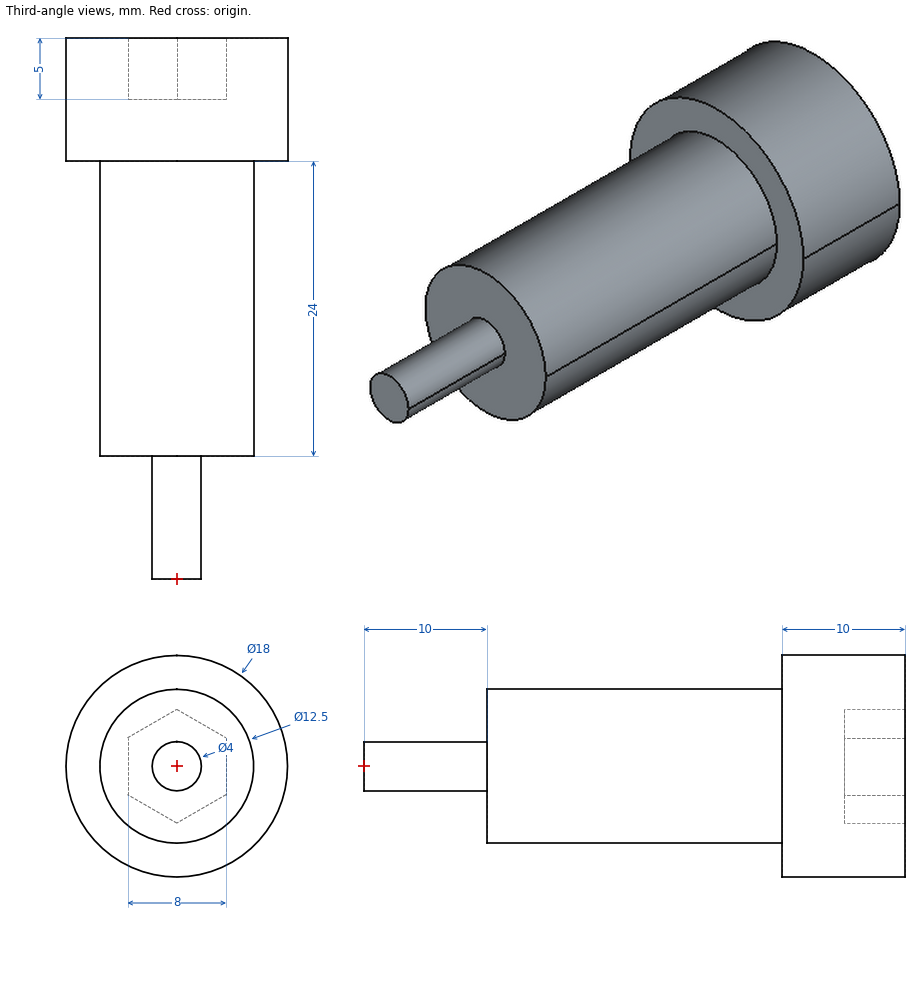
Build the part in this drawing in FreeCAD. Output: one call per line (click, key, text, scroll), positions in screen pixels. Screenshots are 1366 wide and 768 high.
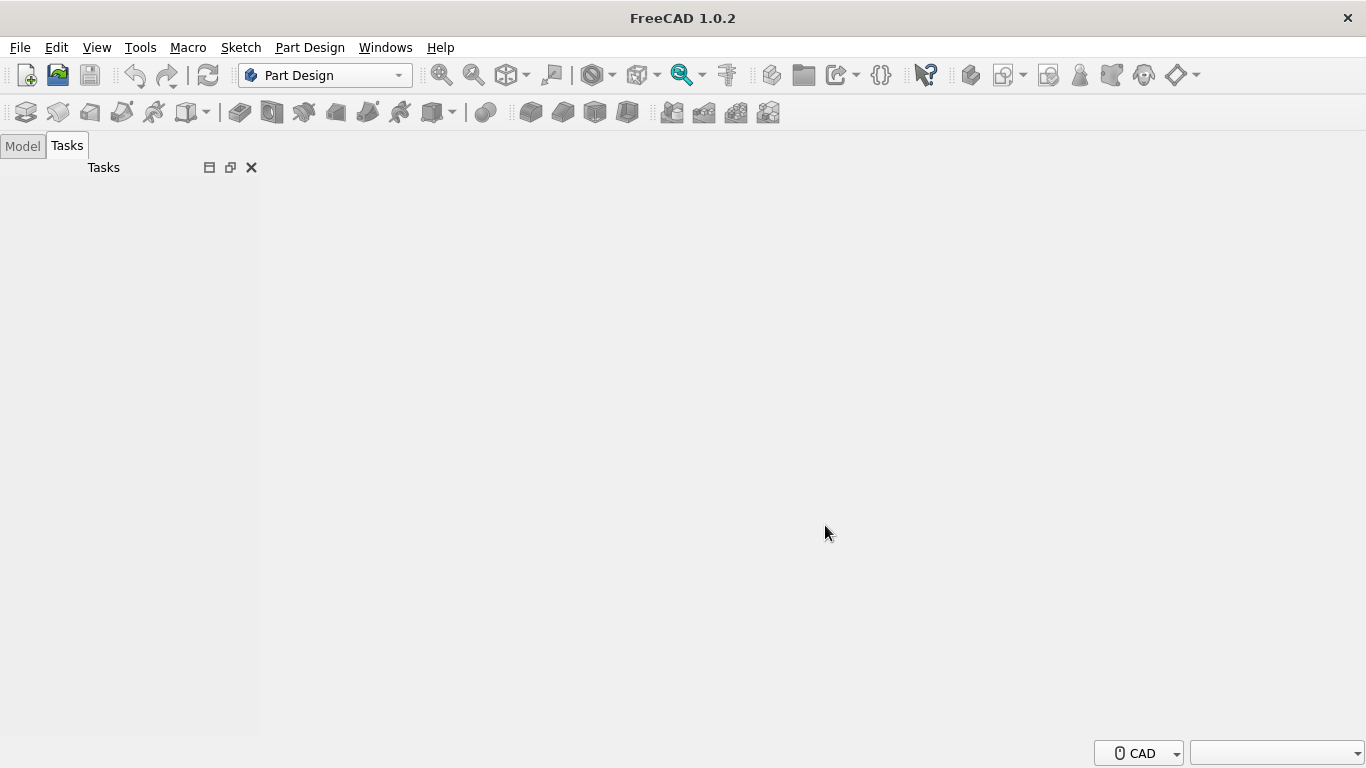
key(ctrl+n)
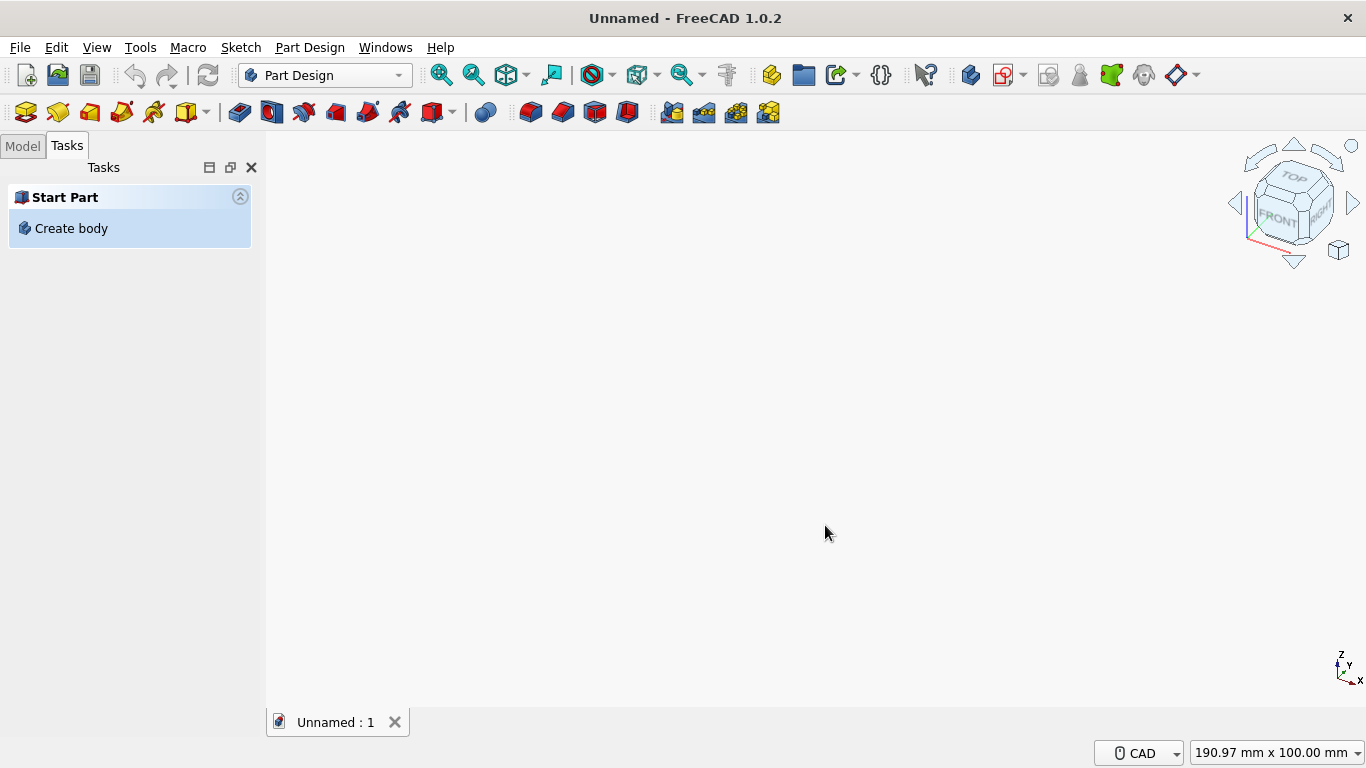
click(1004, 76)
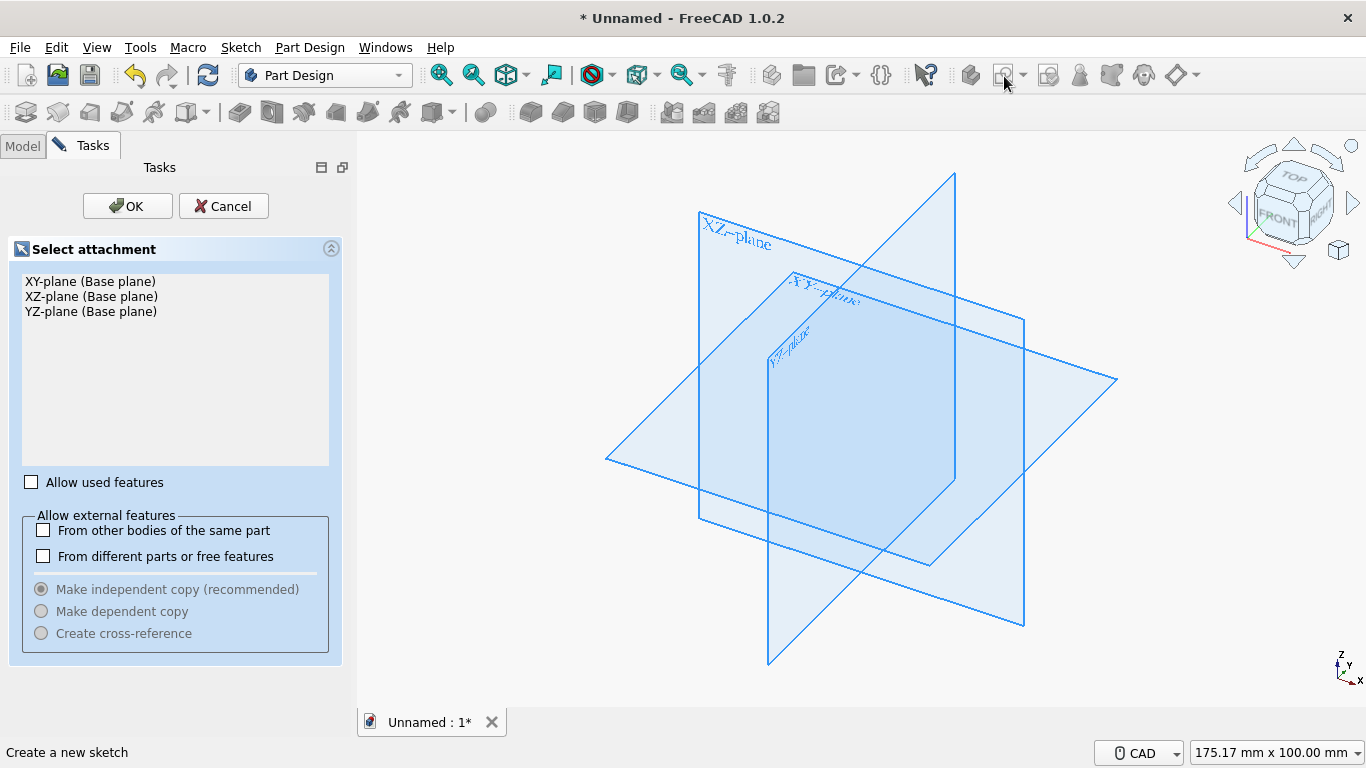
click(82, 296)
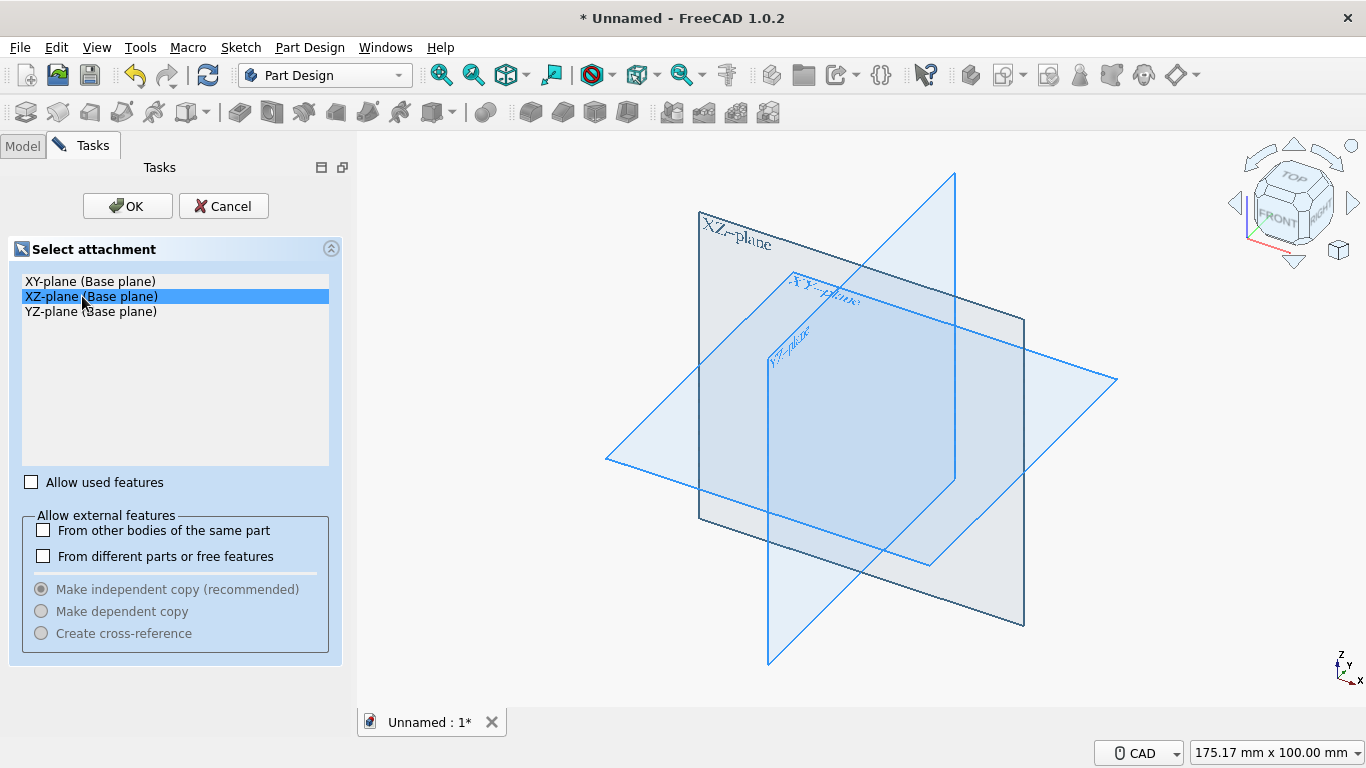
click(128, 206)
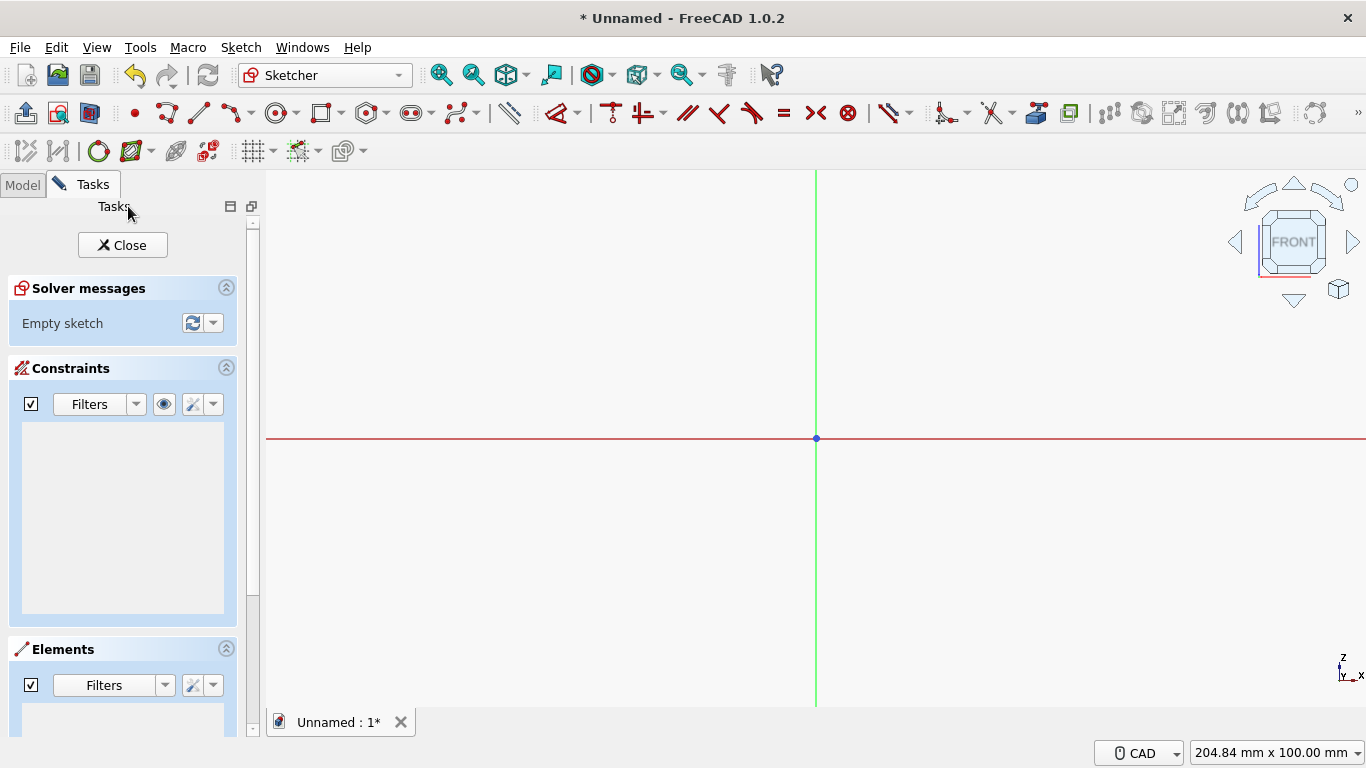
scroll(820, 438, up, 14)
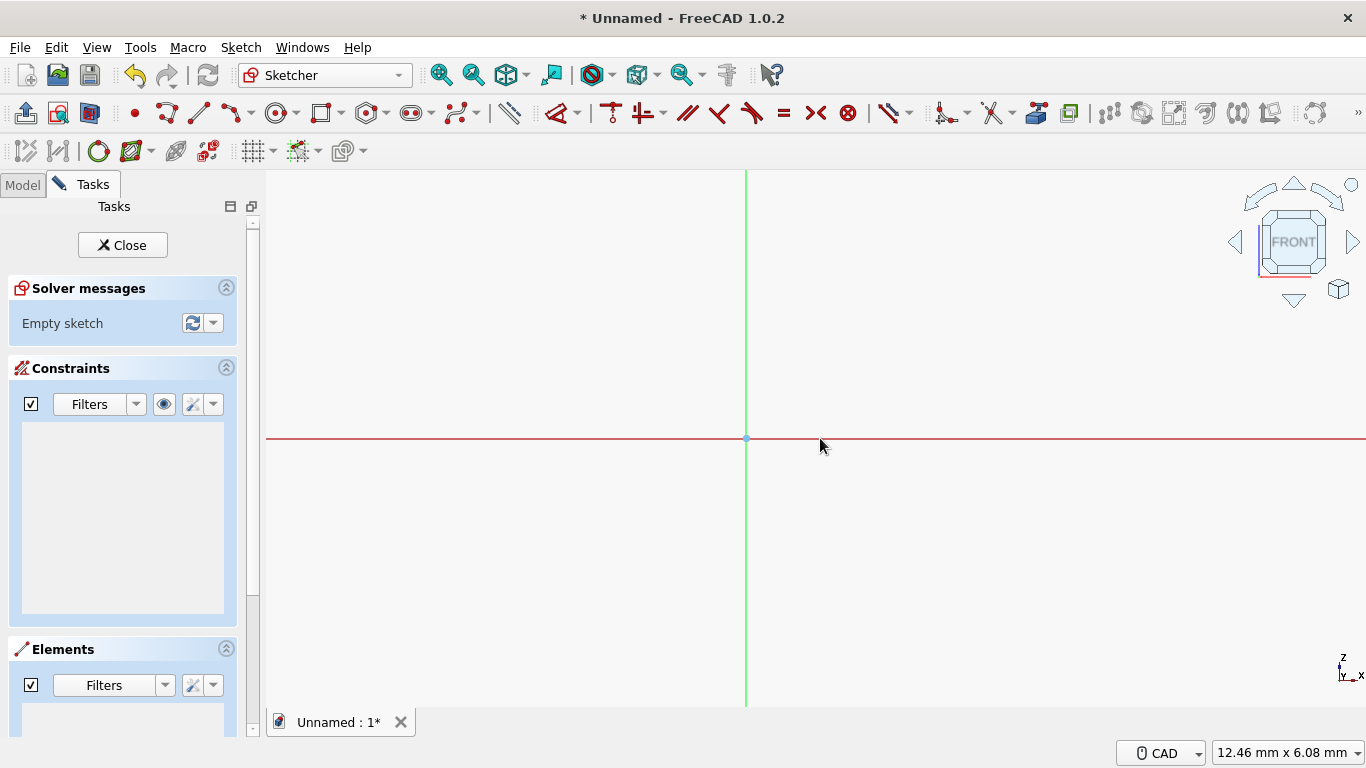
key(g)
key(c)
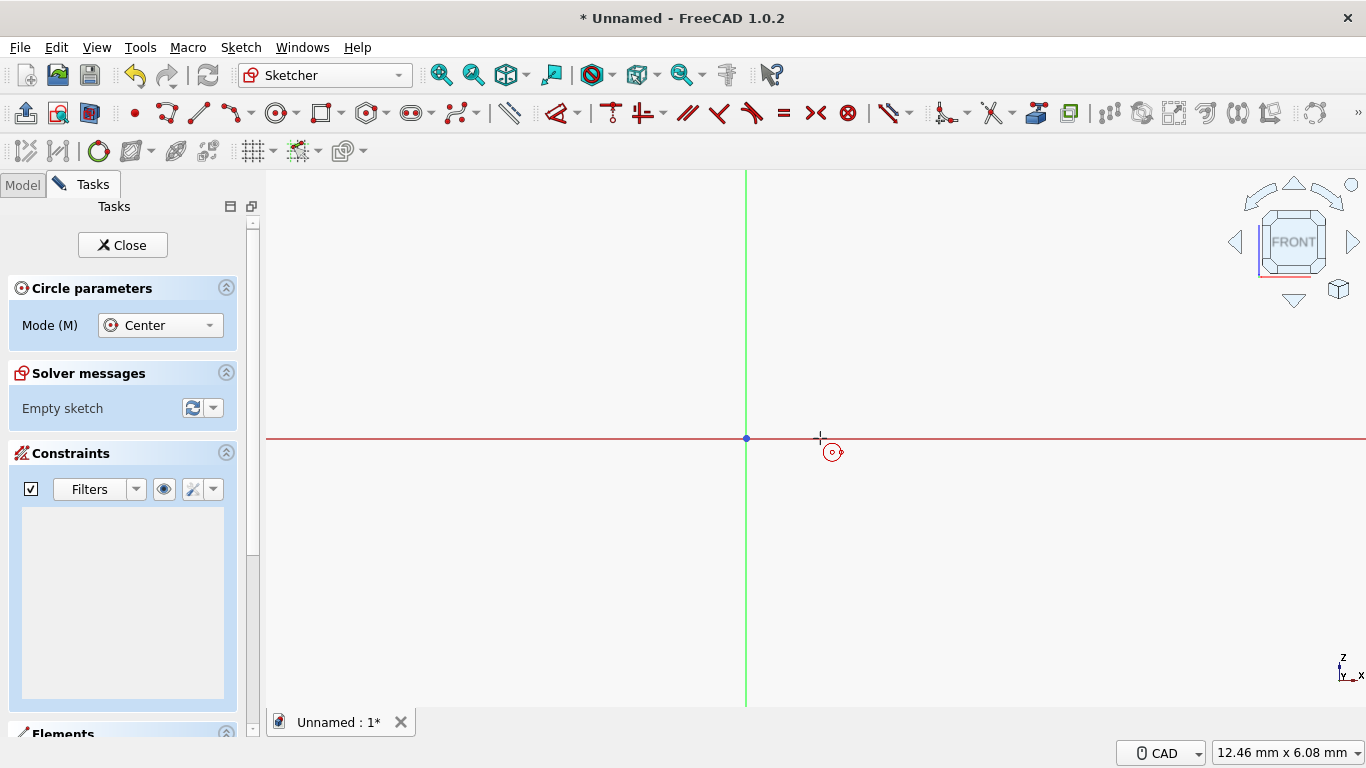
click(746, 438)
move(871, 314)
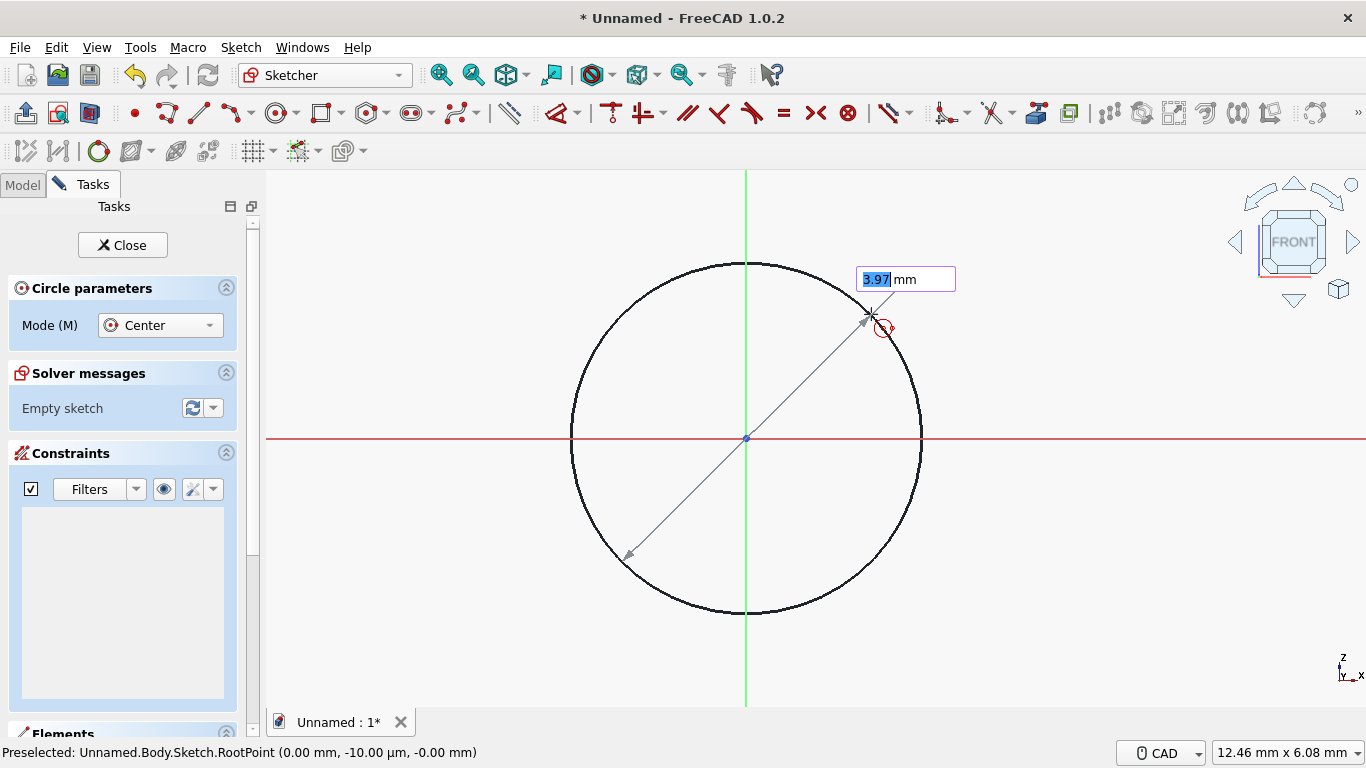
text(4)
key(Return)
key(Escape)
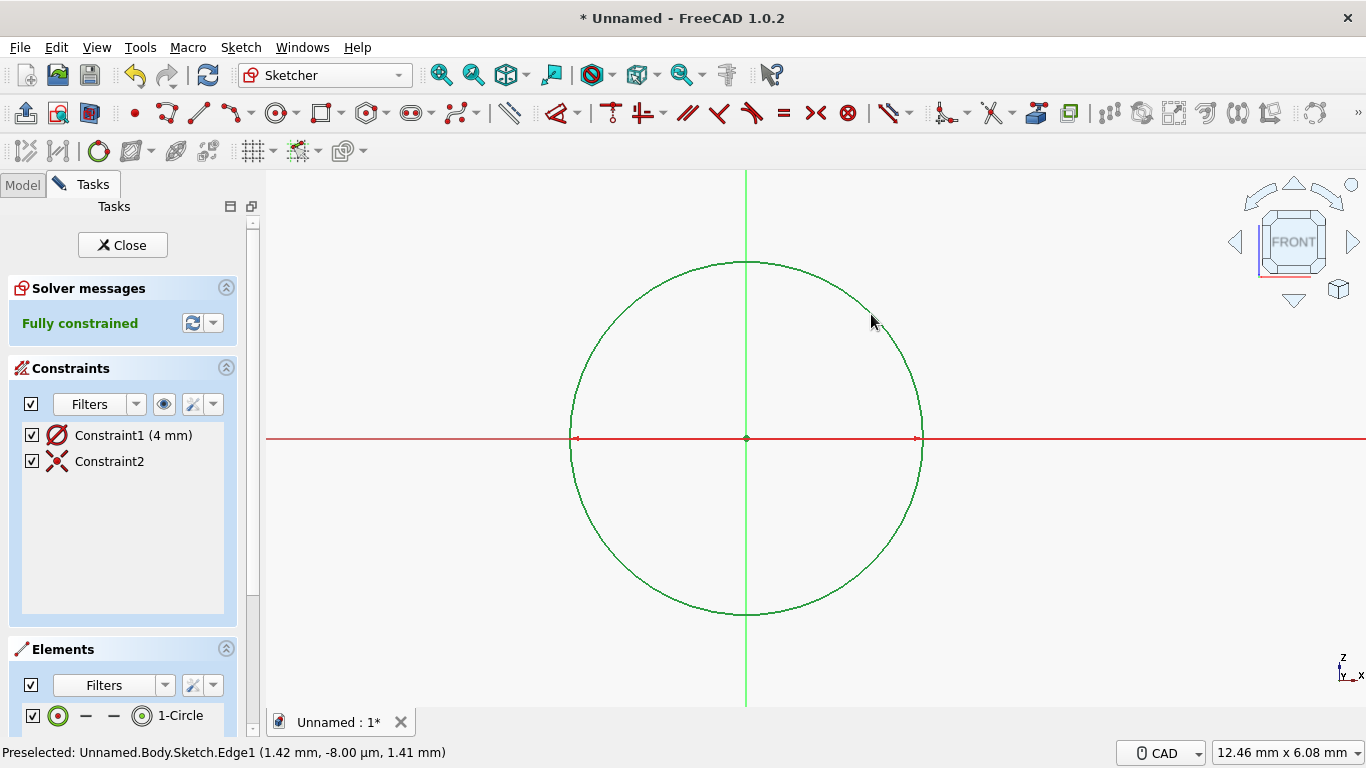
click(123, 245)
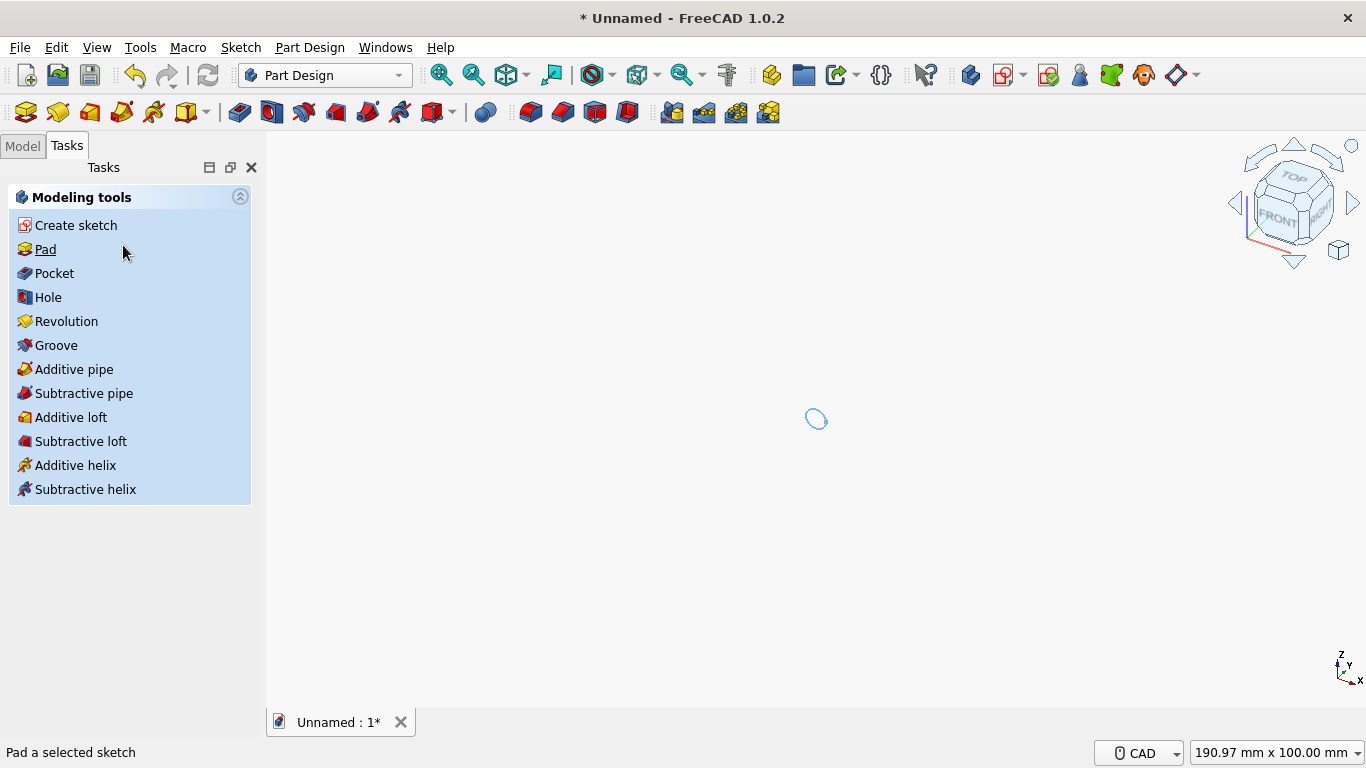
click(26, 112)